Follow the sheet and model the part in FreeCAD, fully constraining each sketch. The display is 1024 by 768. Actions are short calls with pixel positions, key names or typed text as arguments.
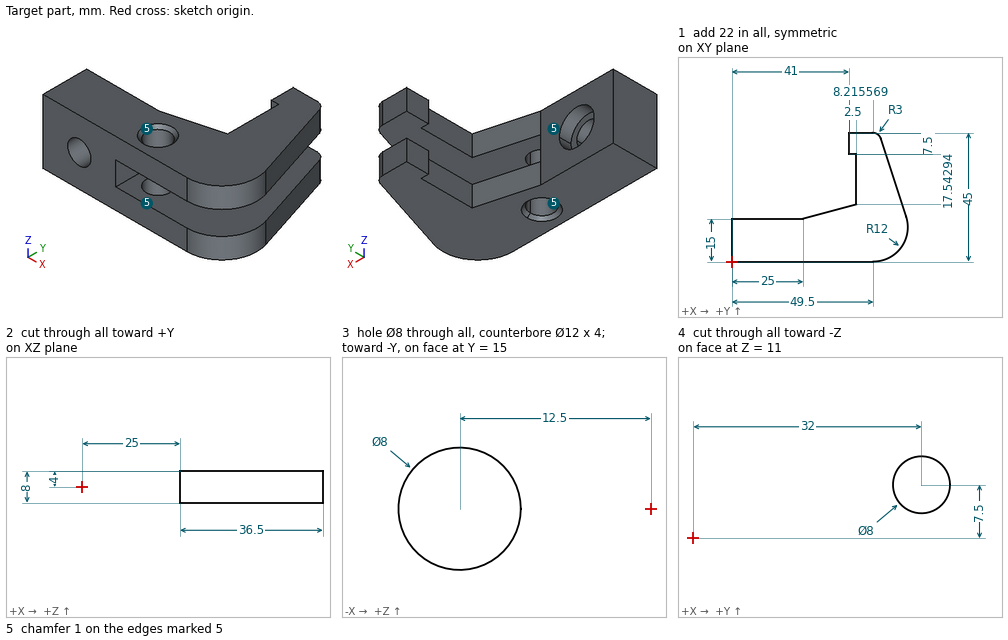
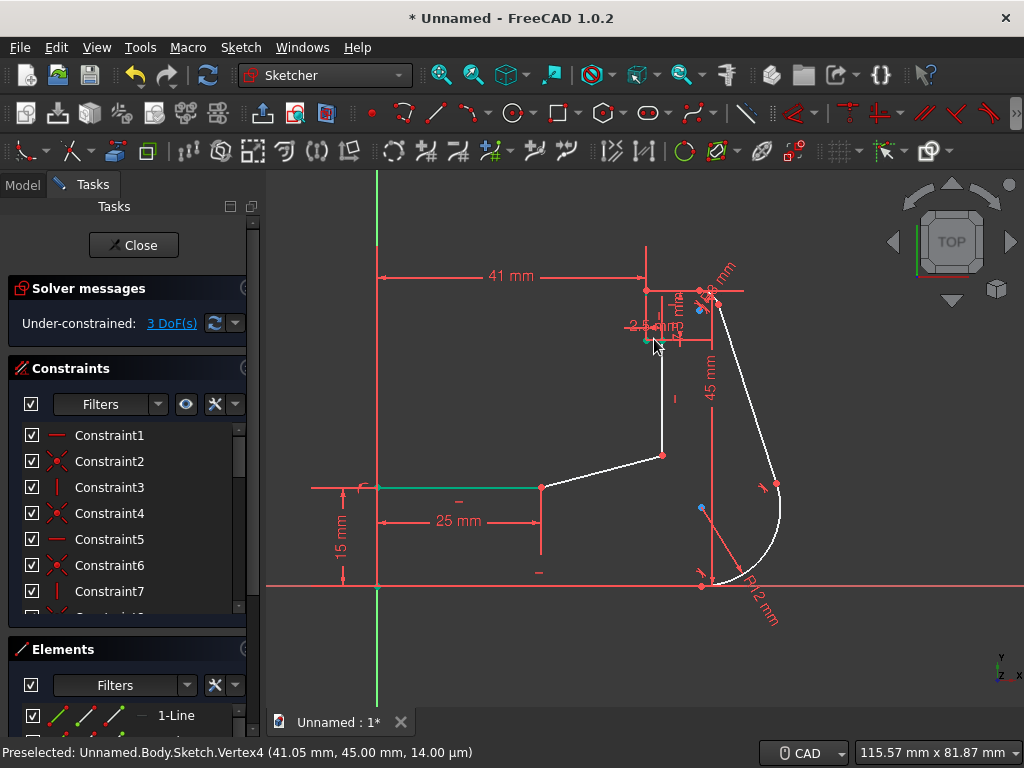
click(474, 586)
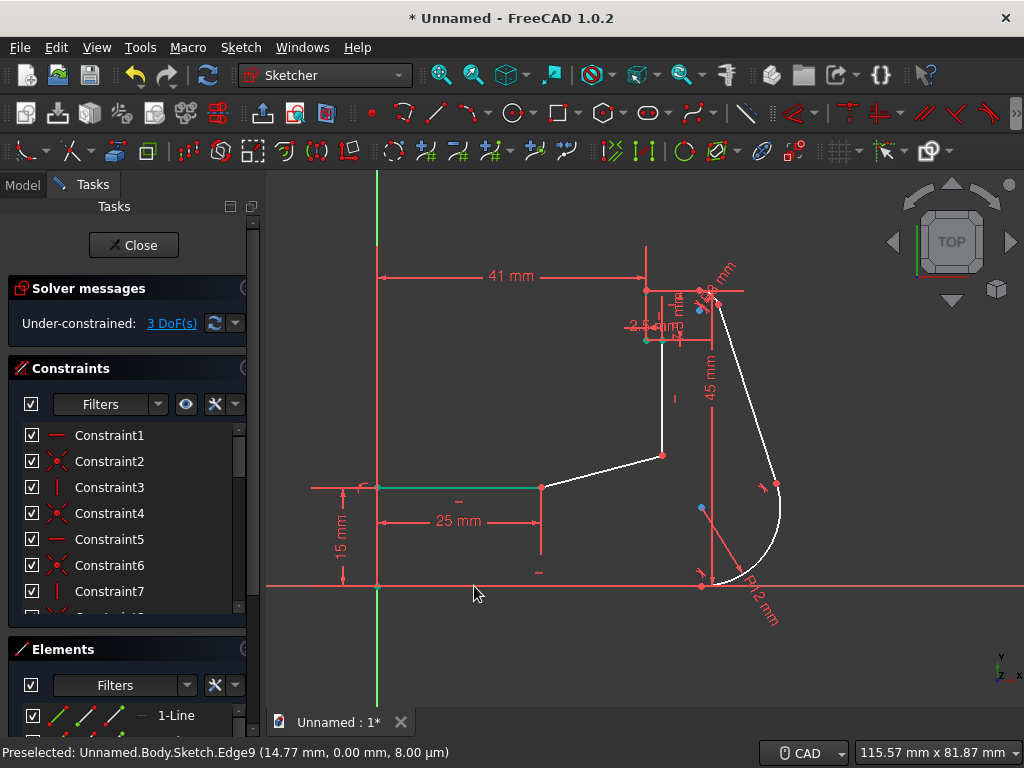
key(l)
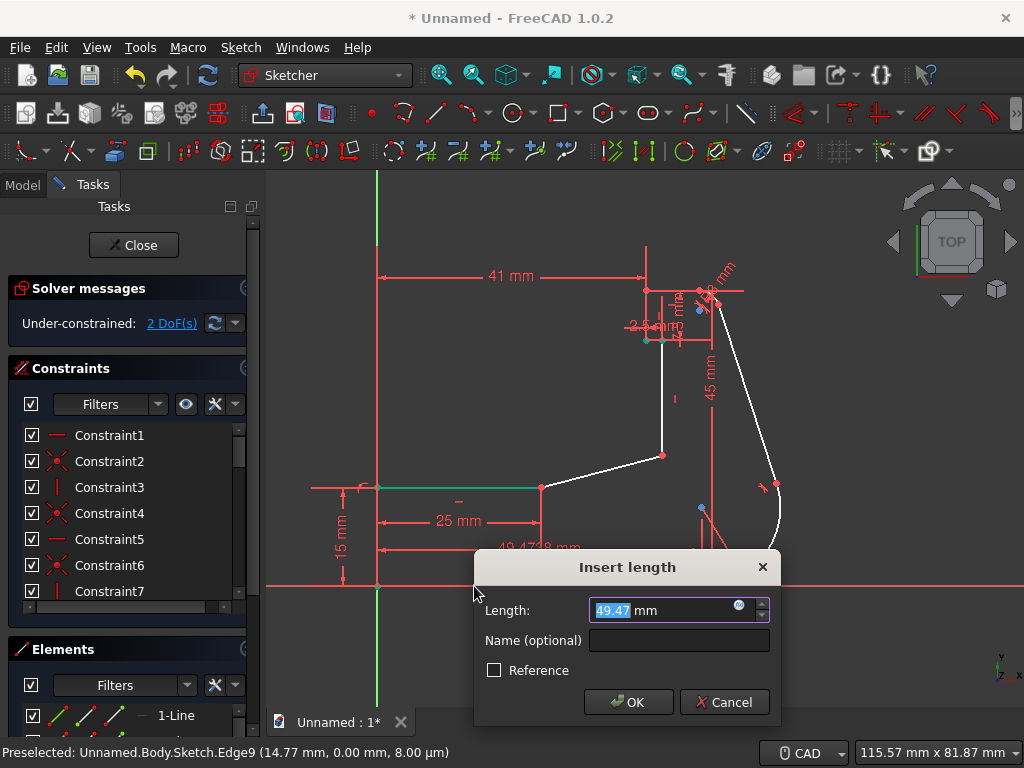
text(49.5)
key(Return)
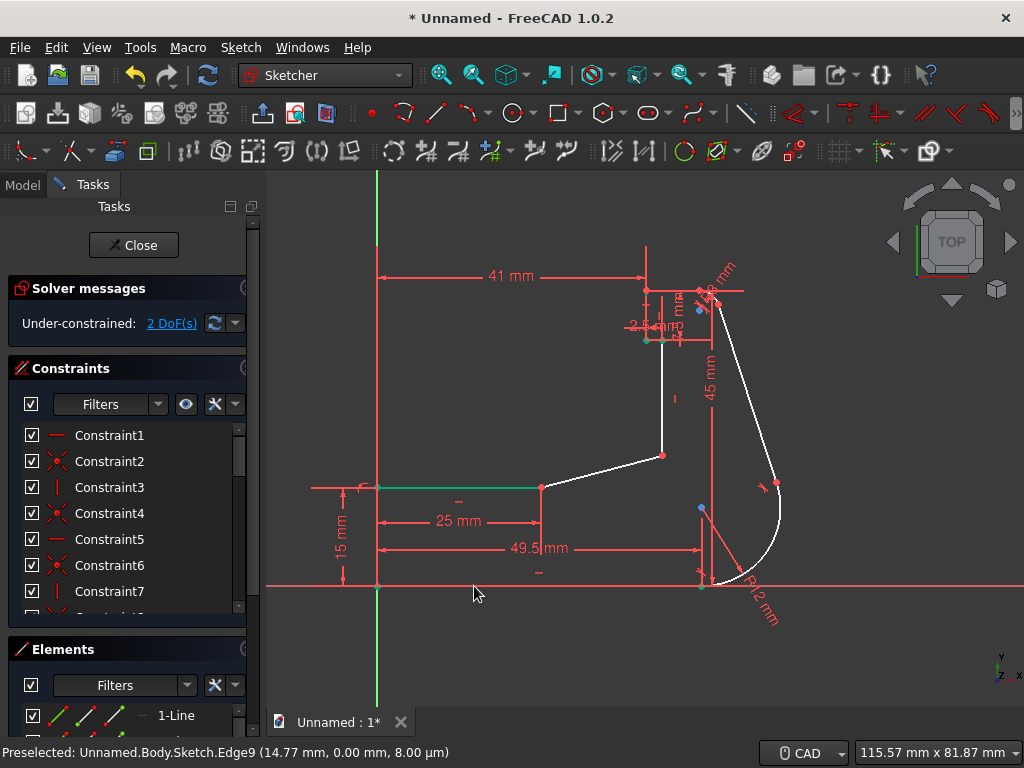
click(662, 291)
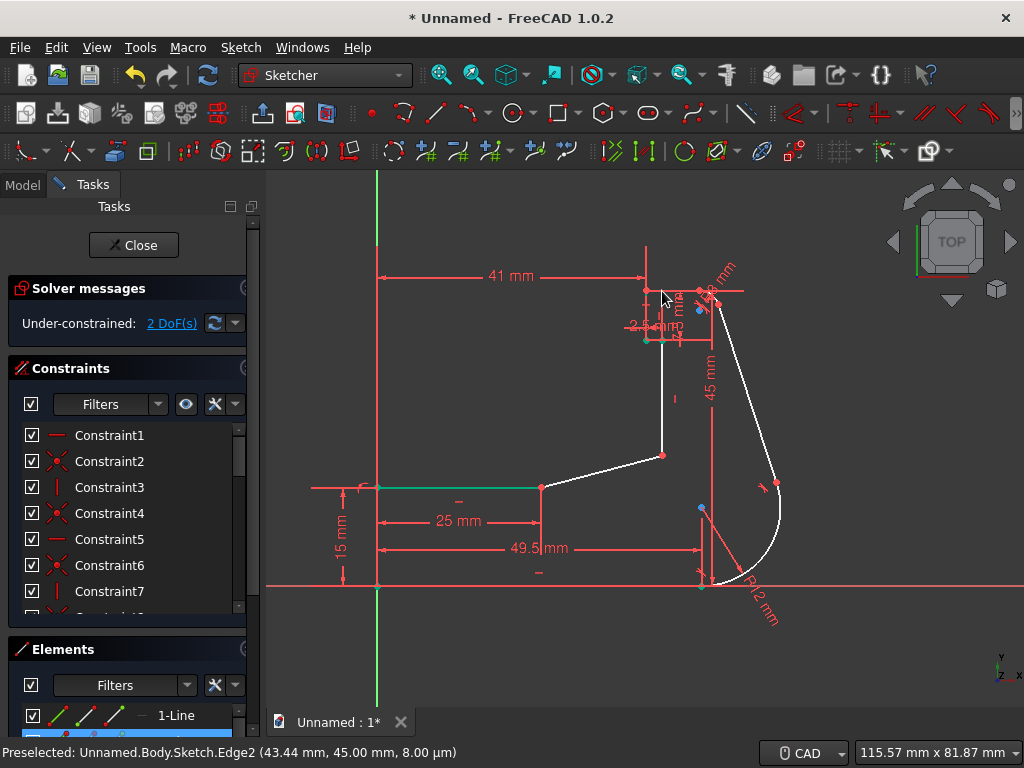
key(l)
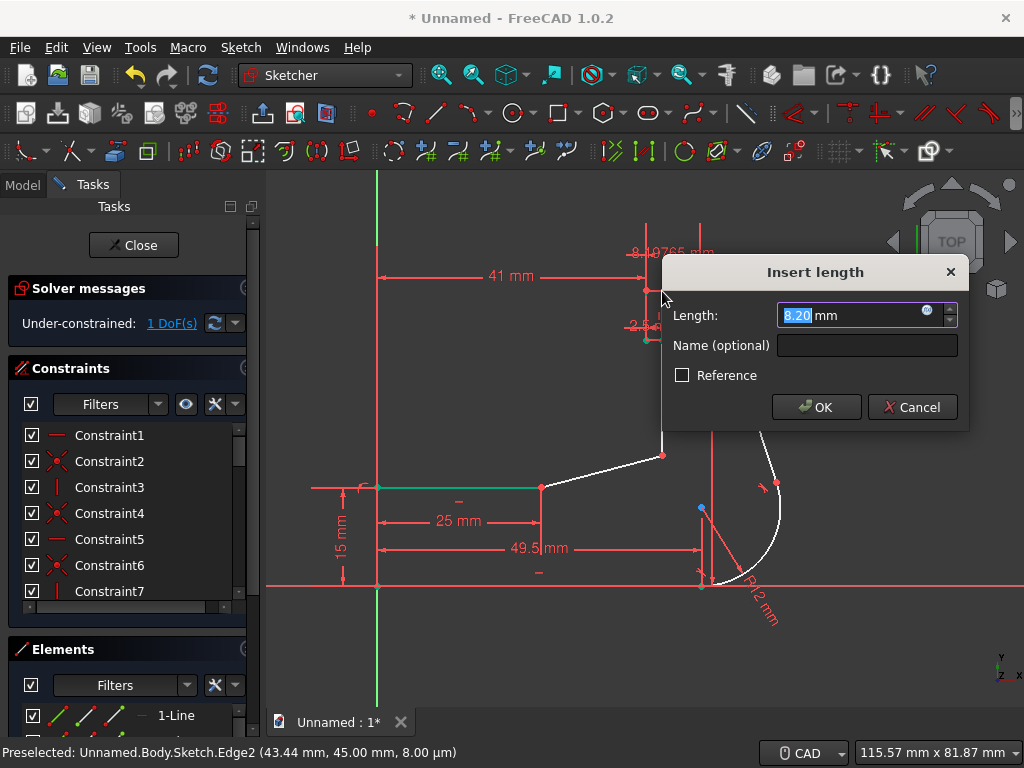
text(8.215569)
key(Return)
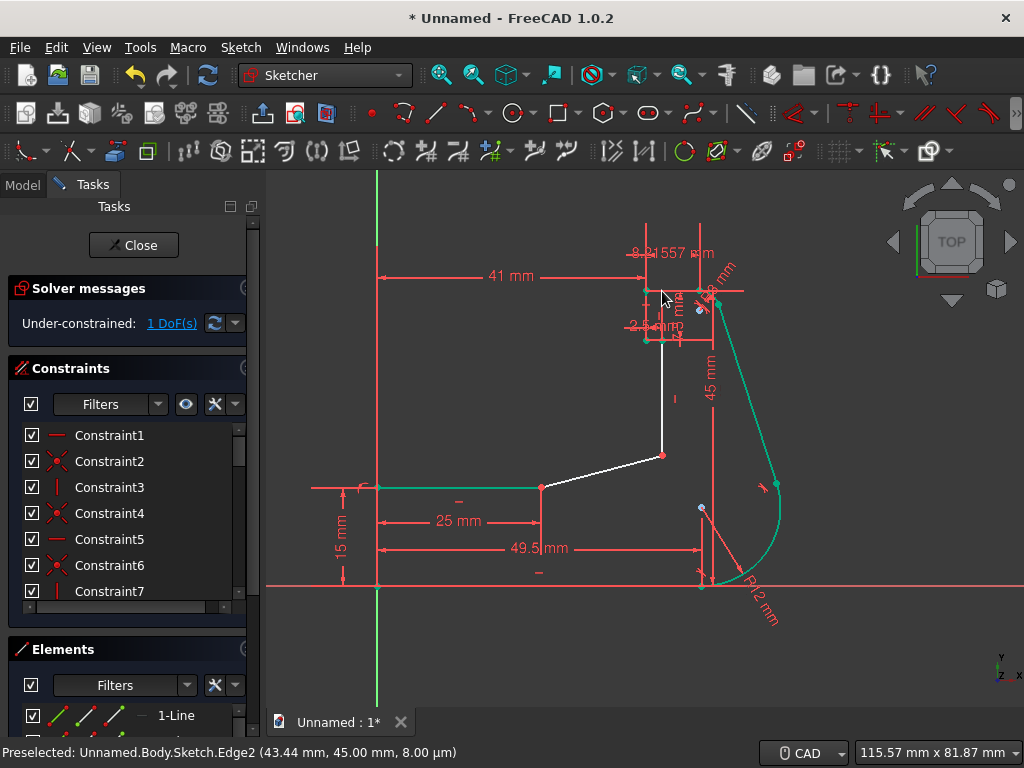
click(662, 375)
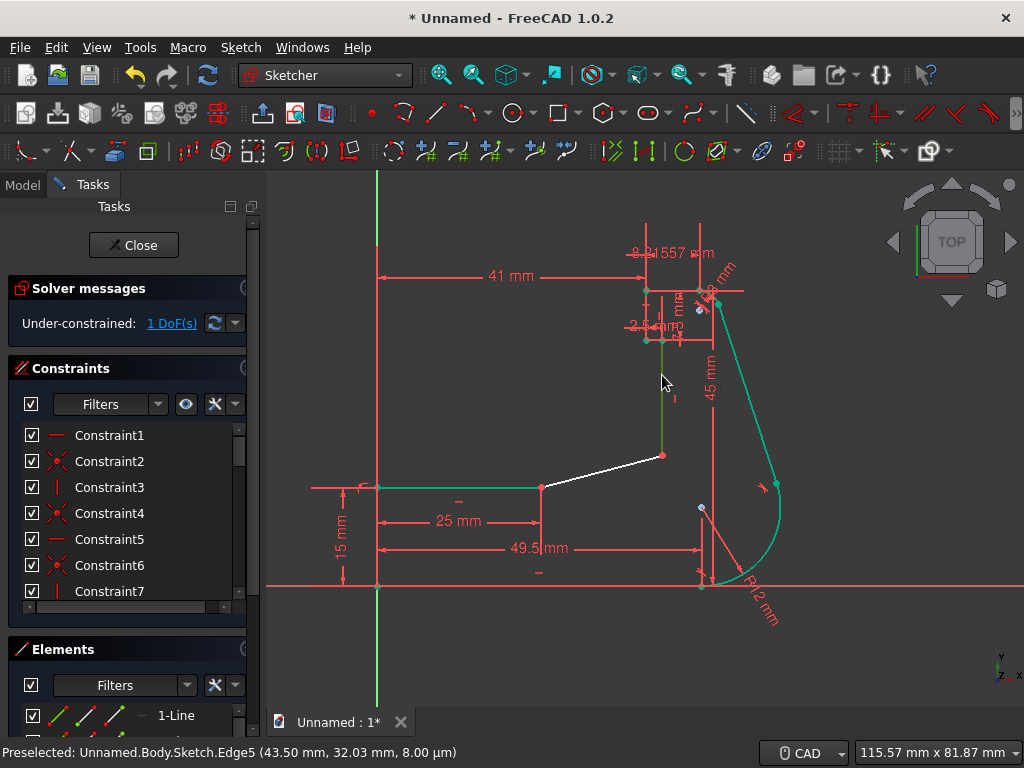
key(i)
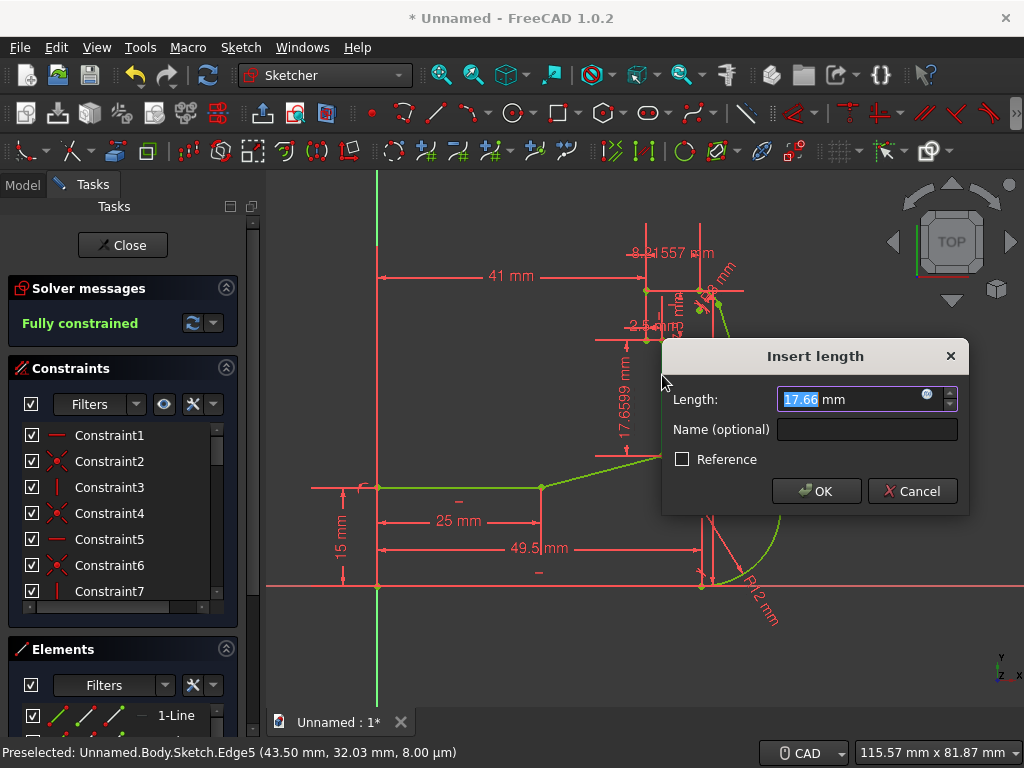
text(17.54294)
key(Return)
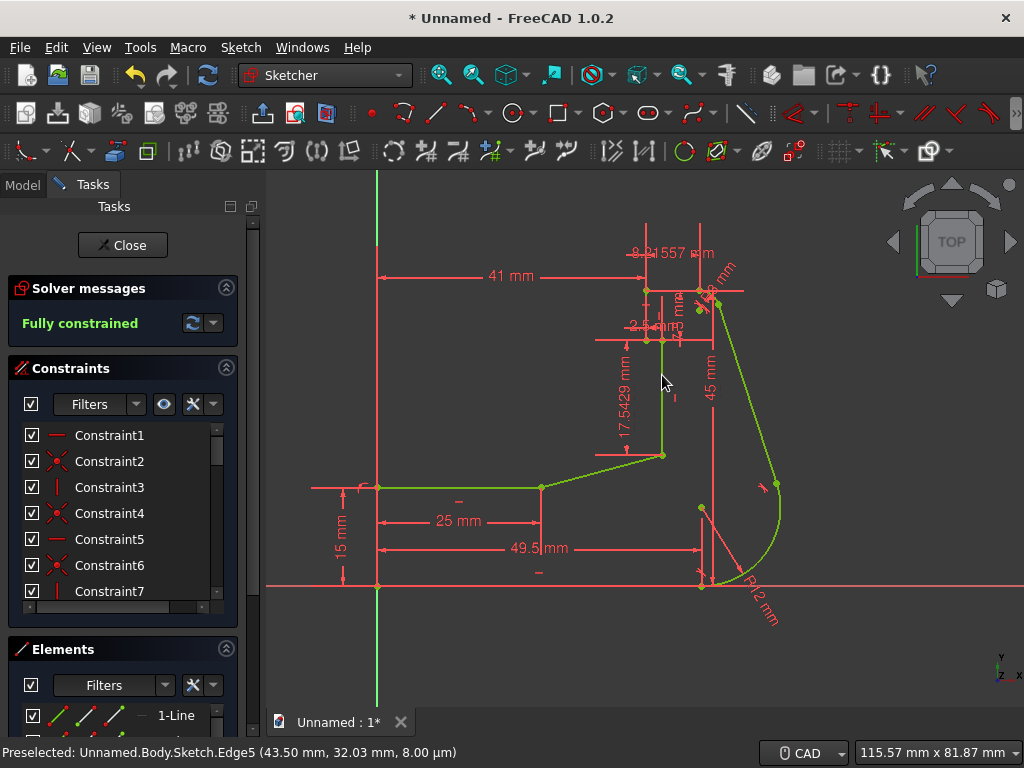
click(123, 245)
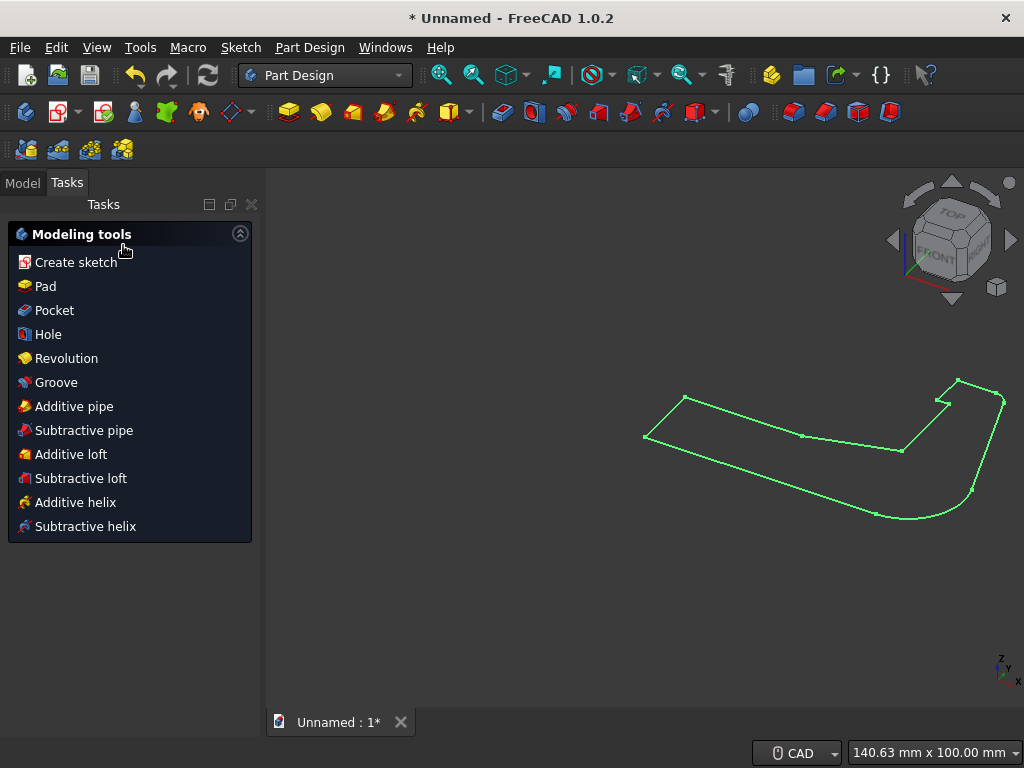
click(290, 112)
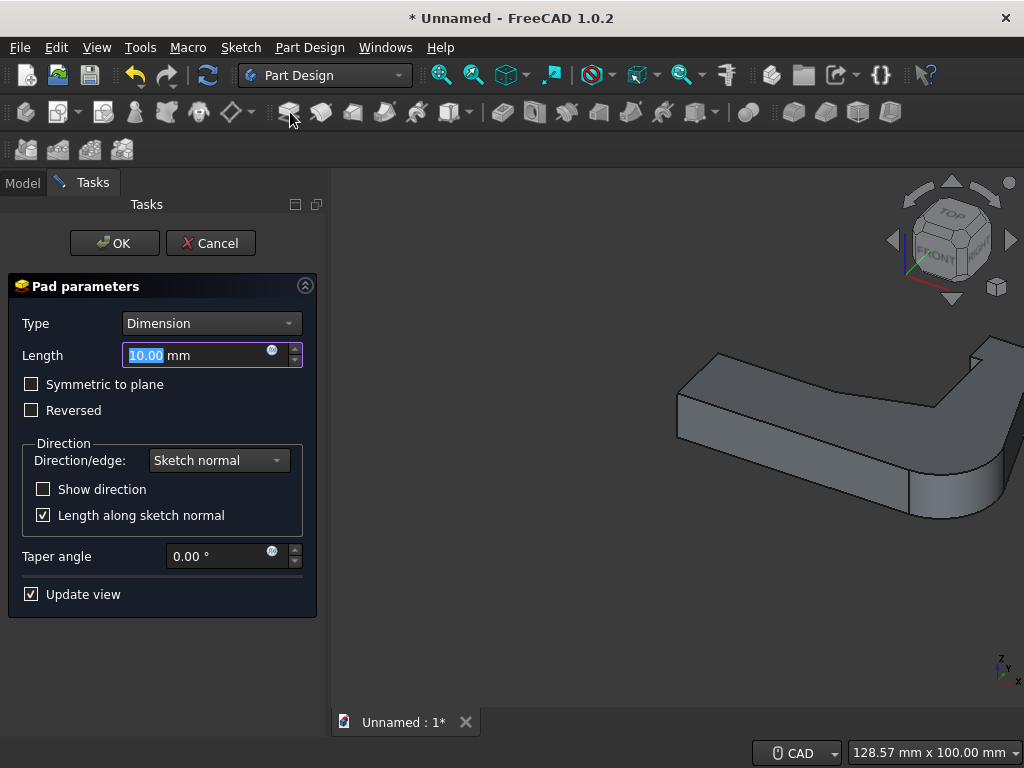
text(22)
key(Tab)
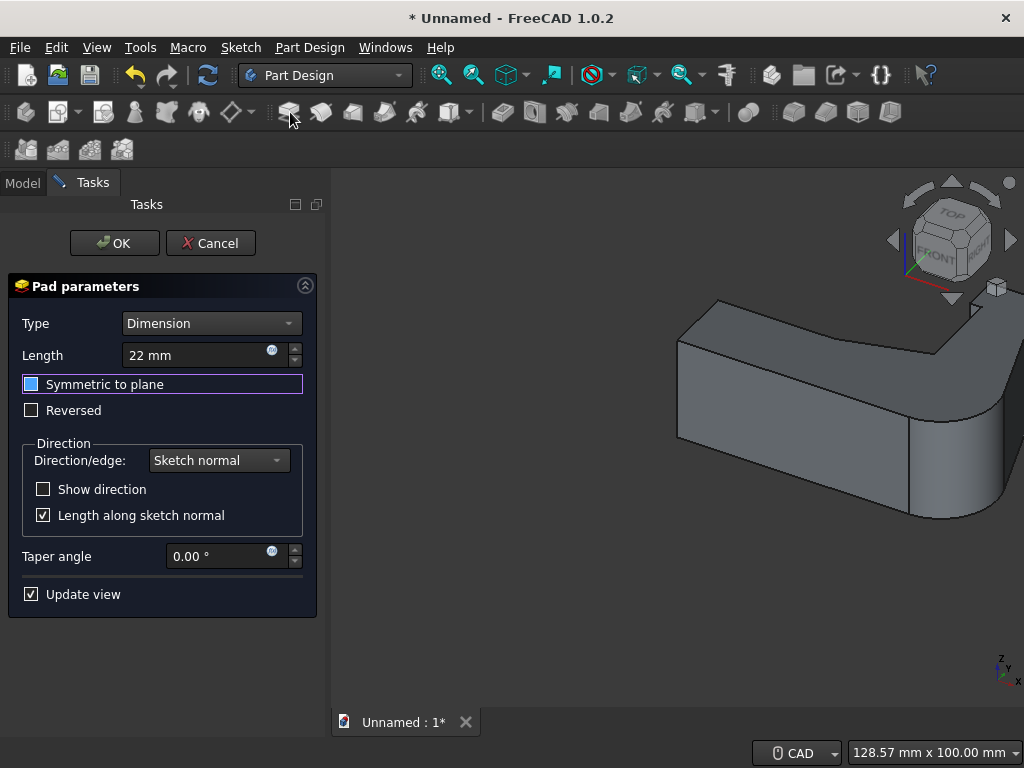
click(30, 384)